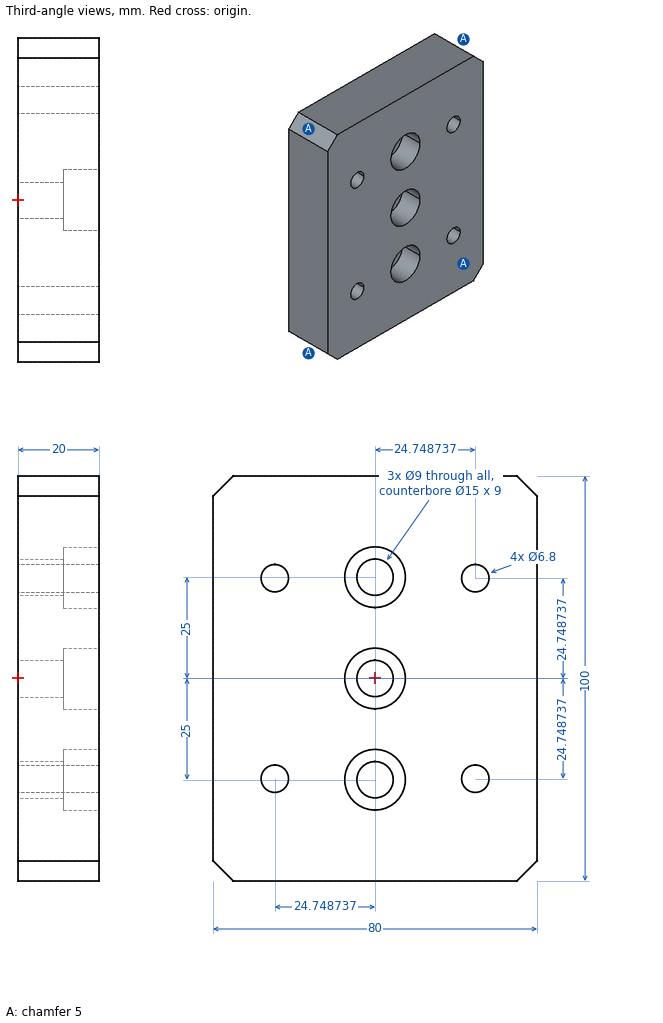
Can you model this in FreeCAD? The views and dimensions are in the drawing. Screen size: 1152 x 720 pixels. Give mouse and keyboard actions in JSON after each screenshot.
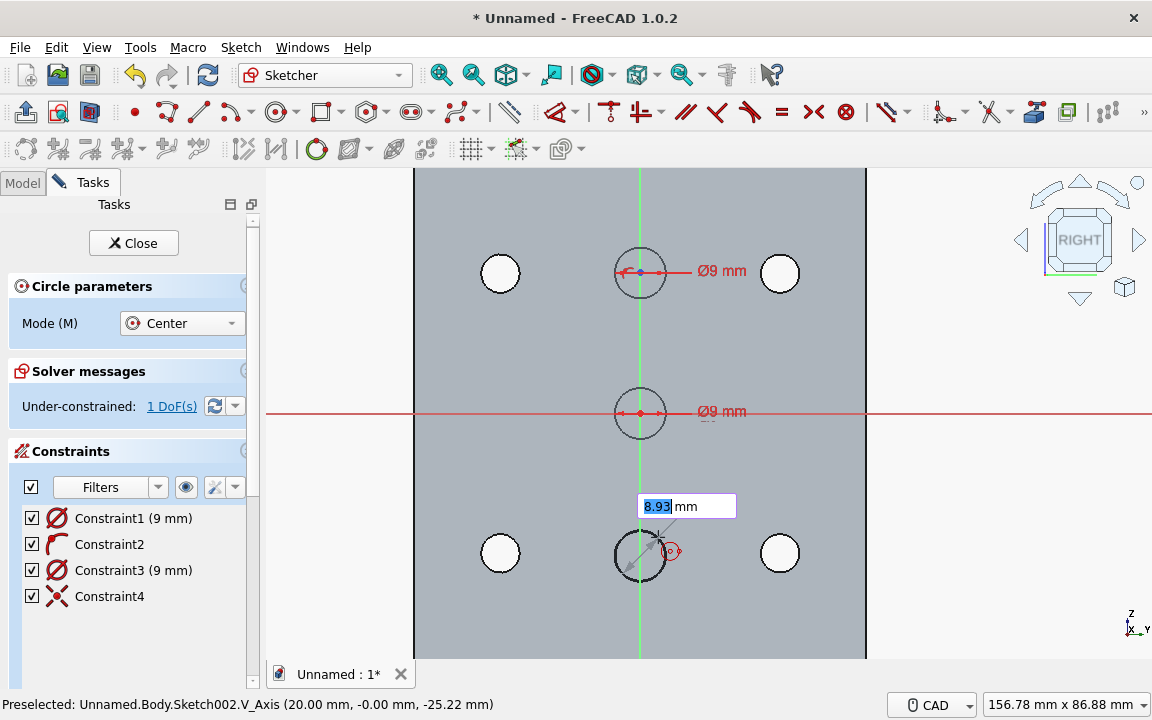
{"action": "type", "text": "9"}
{"action": "key", "text": "Return"}
{"action": "key", "text": "Escape"}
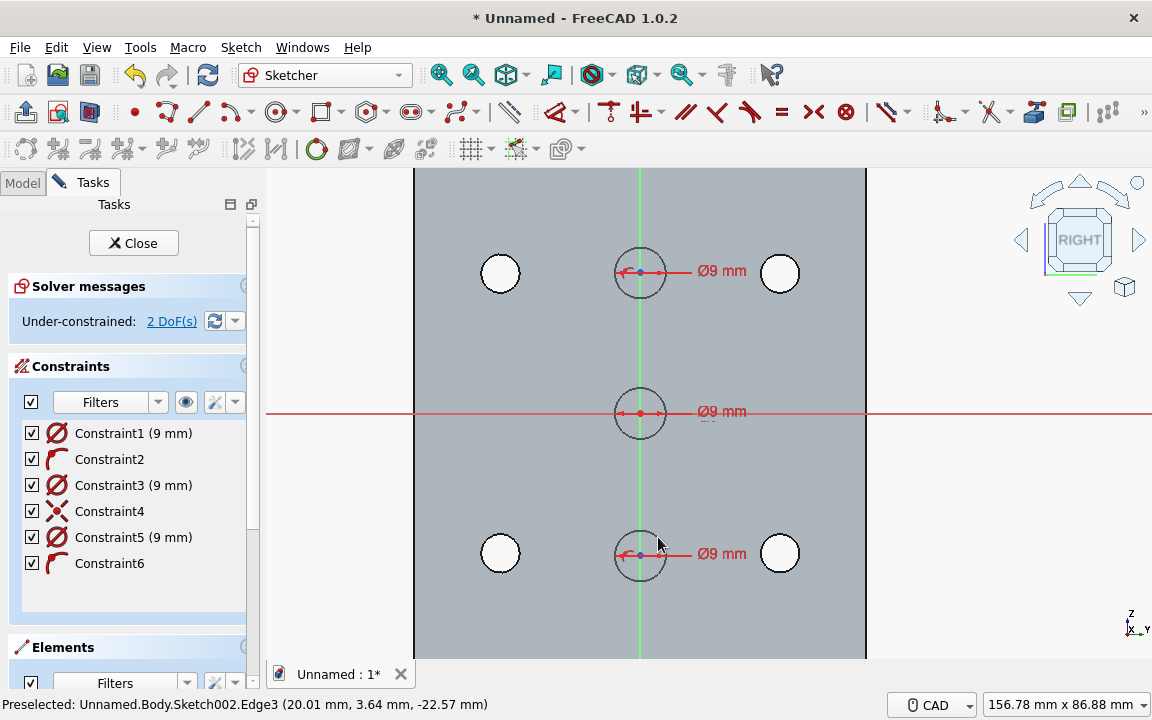
{"action": "key", "text": "d"}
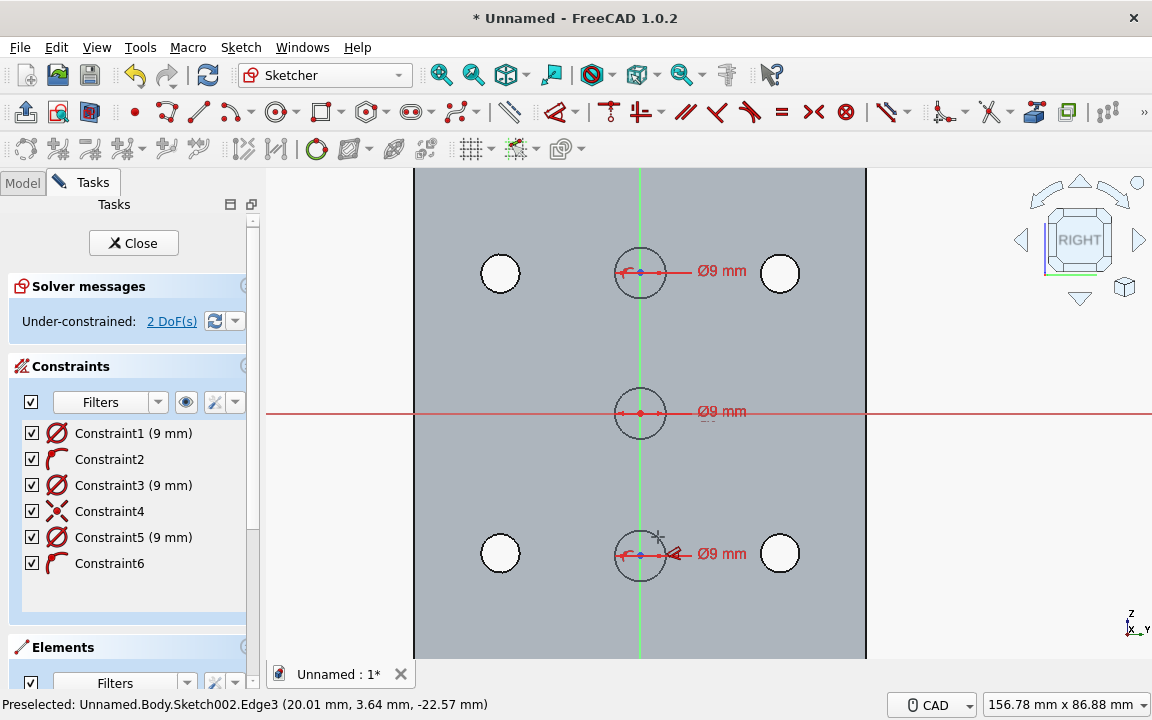
{"action": "left_click", "coordinate": [640, 273]}
{"action": "left_click", "coordinate": [674, 343]}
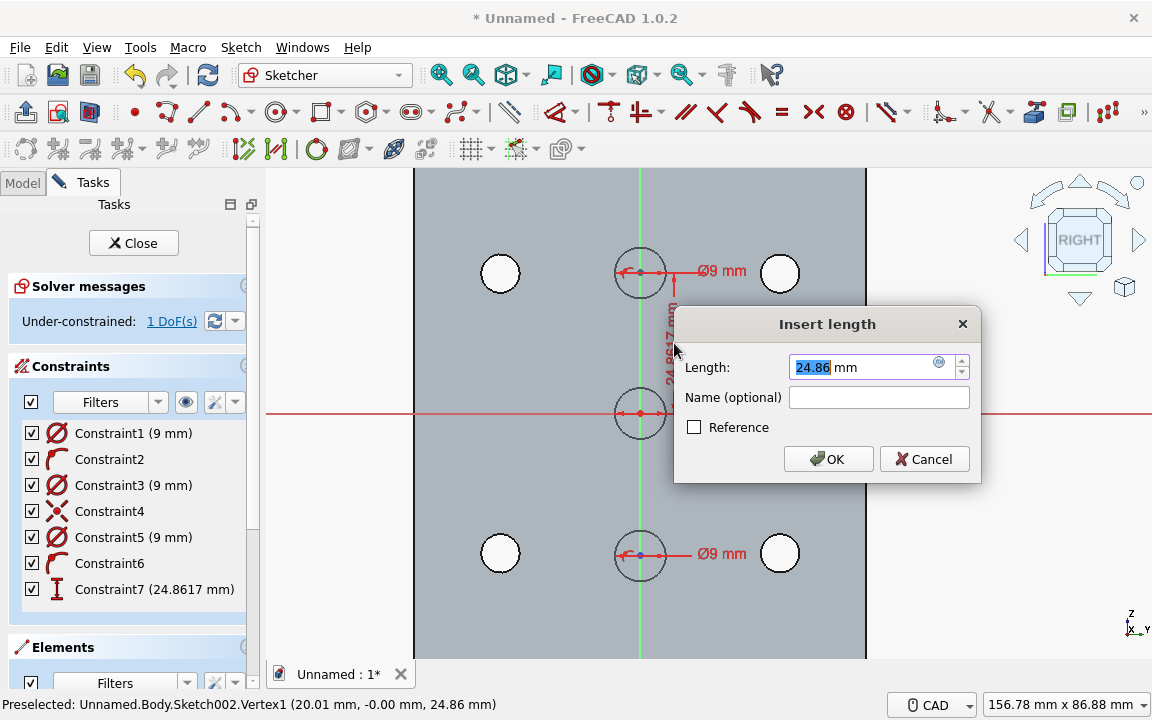
{"action": "type", "text": "25"}
{"action": "key", "text": "Return"}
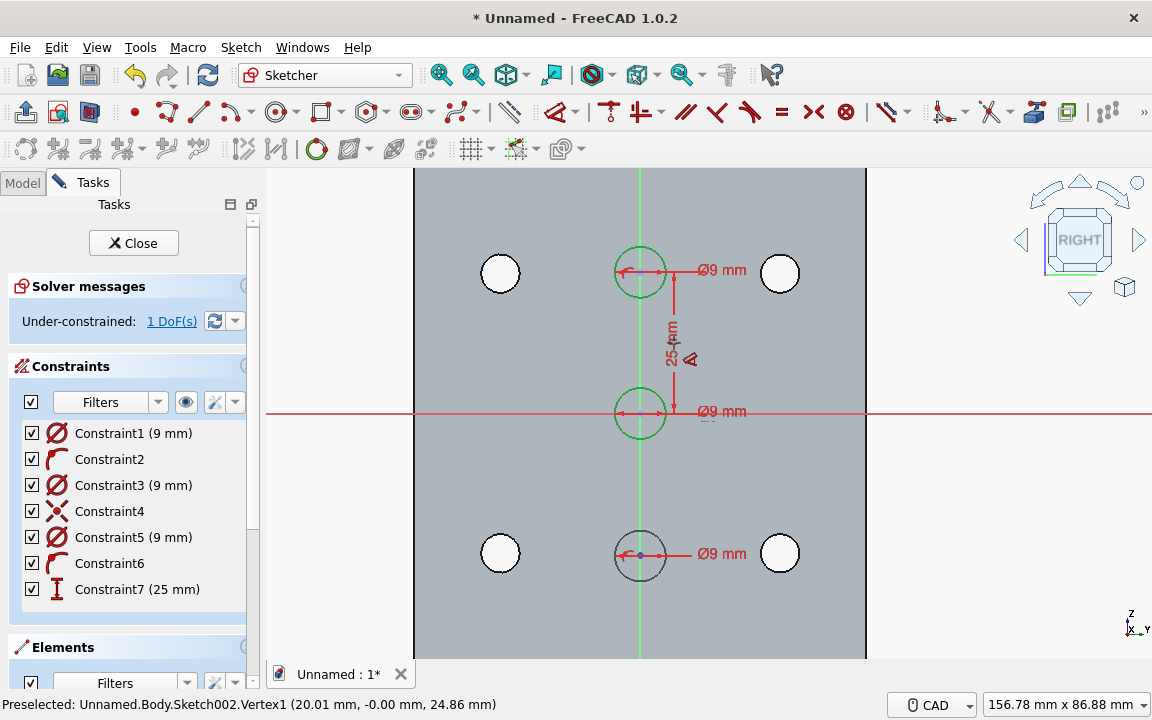
{"action": "left_click", "coordinate": [640, 556]}
{"action": "left_click", "coordinate": [674, 485]}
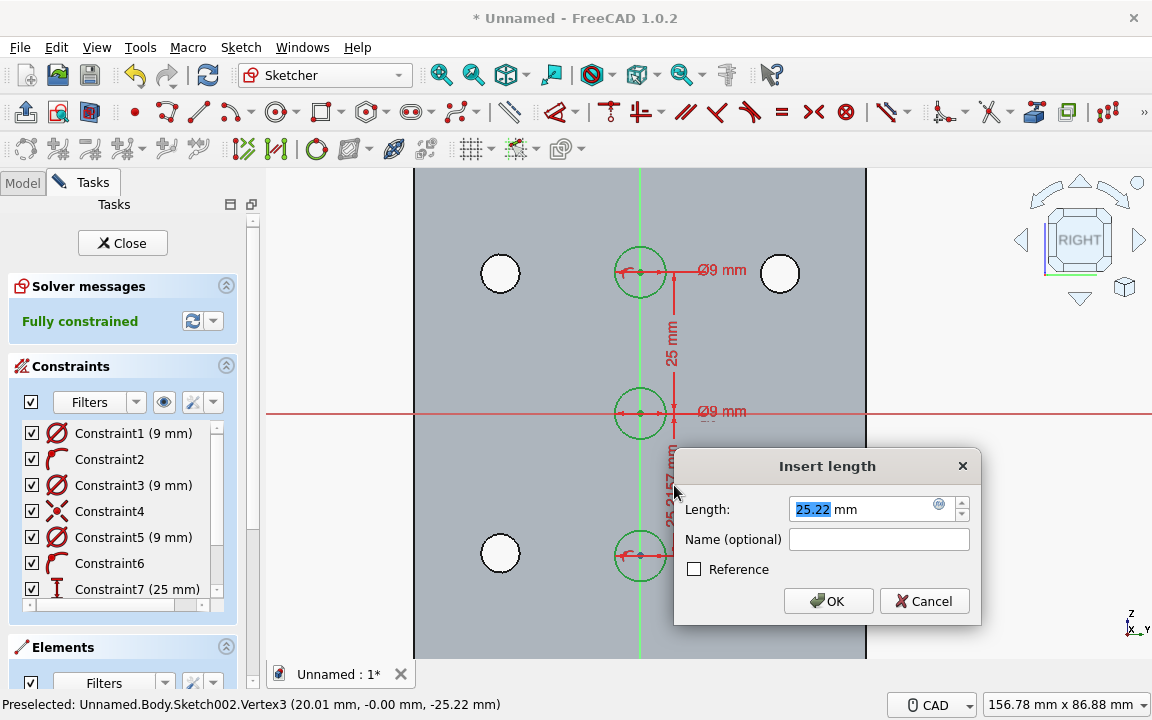
{"action": "type", "text": "25"}
{"action": "key", "text": "Return"}
{"action": "key", "text": "Escape"}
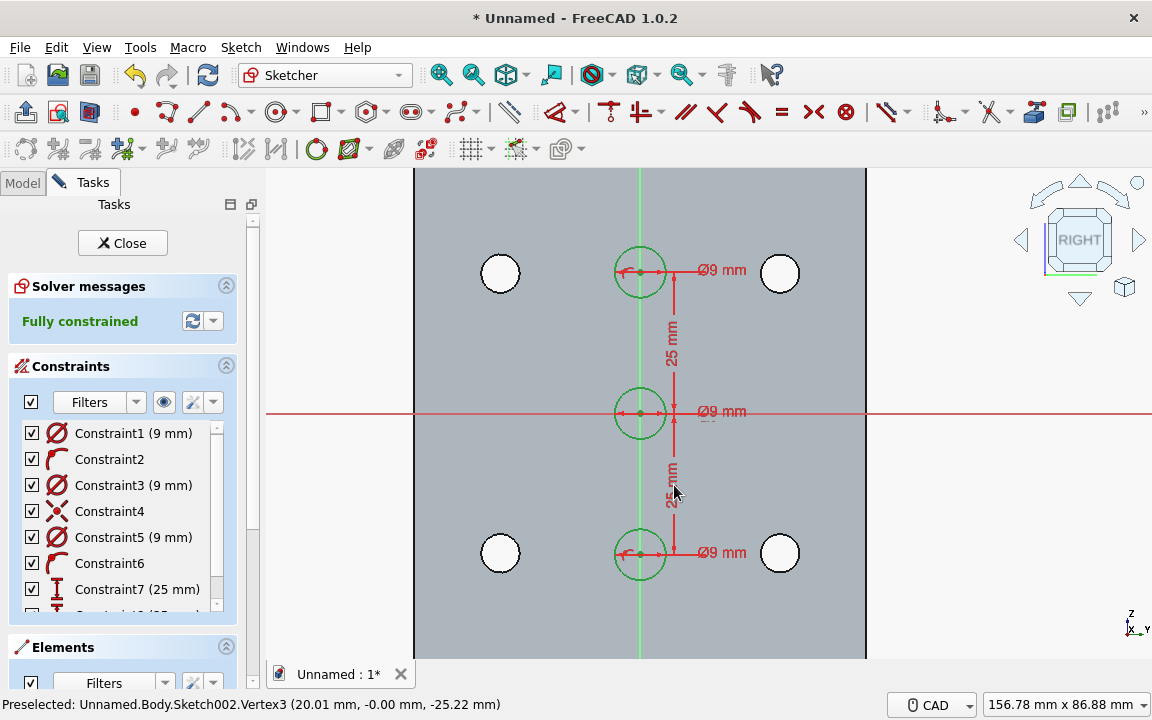
{"action": "left_click", "coordinate": [123, 243]}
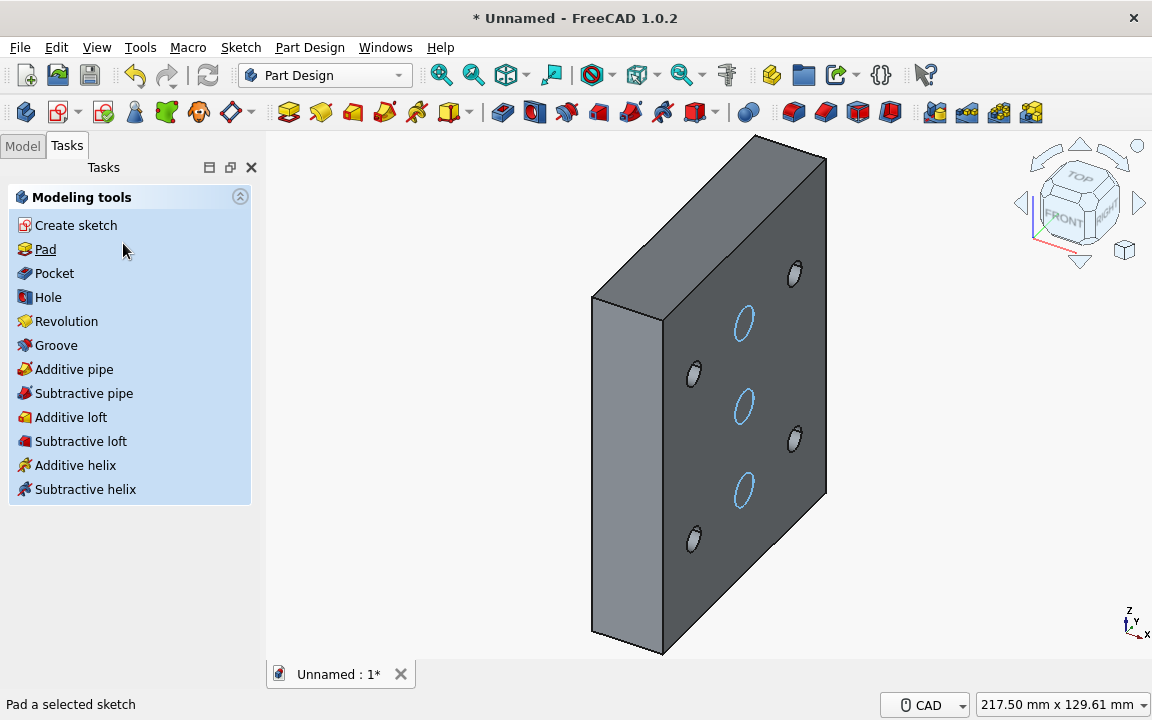
{"action": "left_click", "coordinate": [536, 112]}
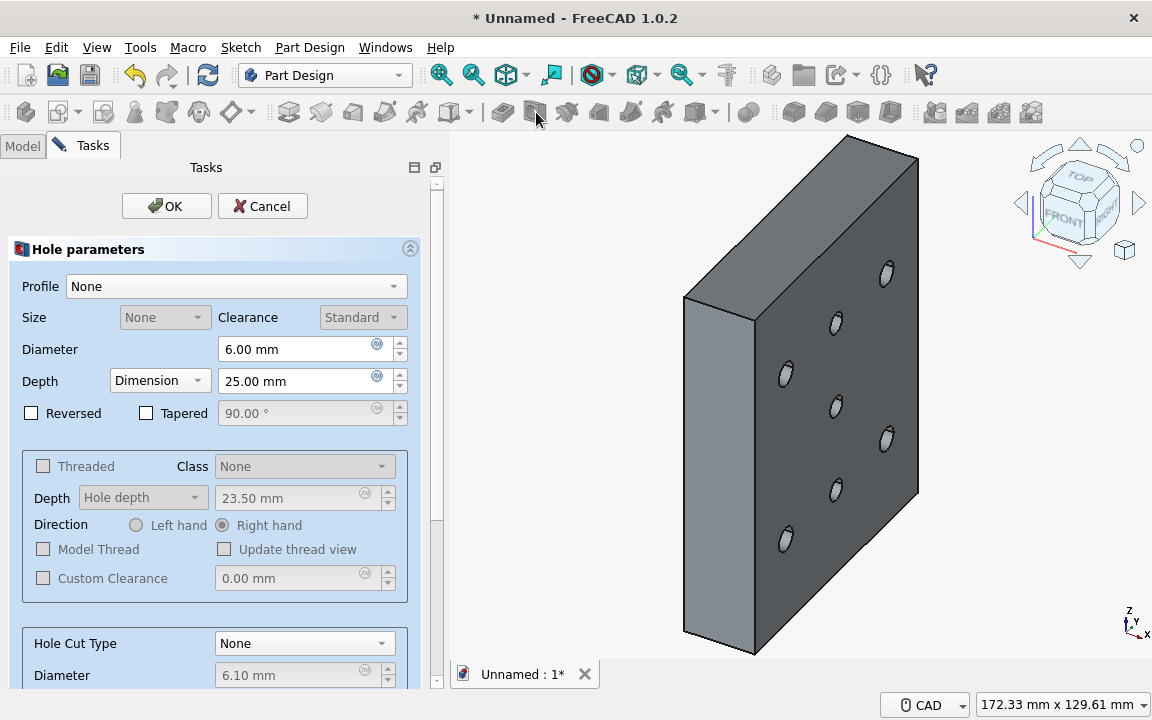
{"action": "triple_click", "coordinate": [305, 349]}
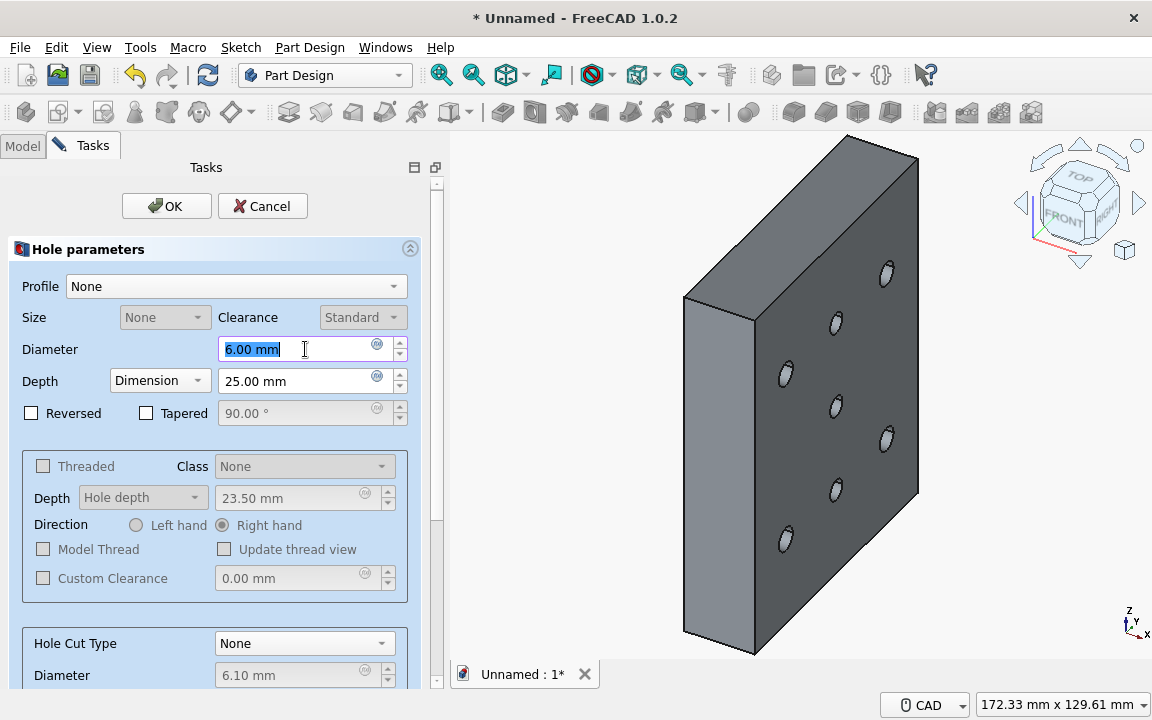
{"action": "type", "text": "9"}
{"action": "key", "text": "Tab"}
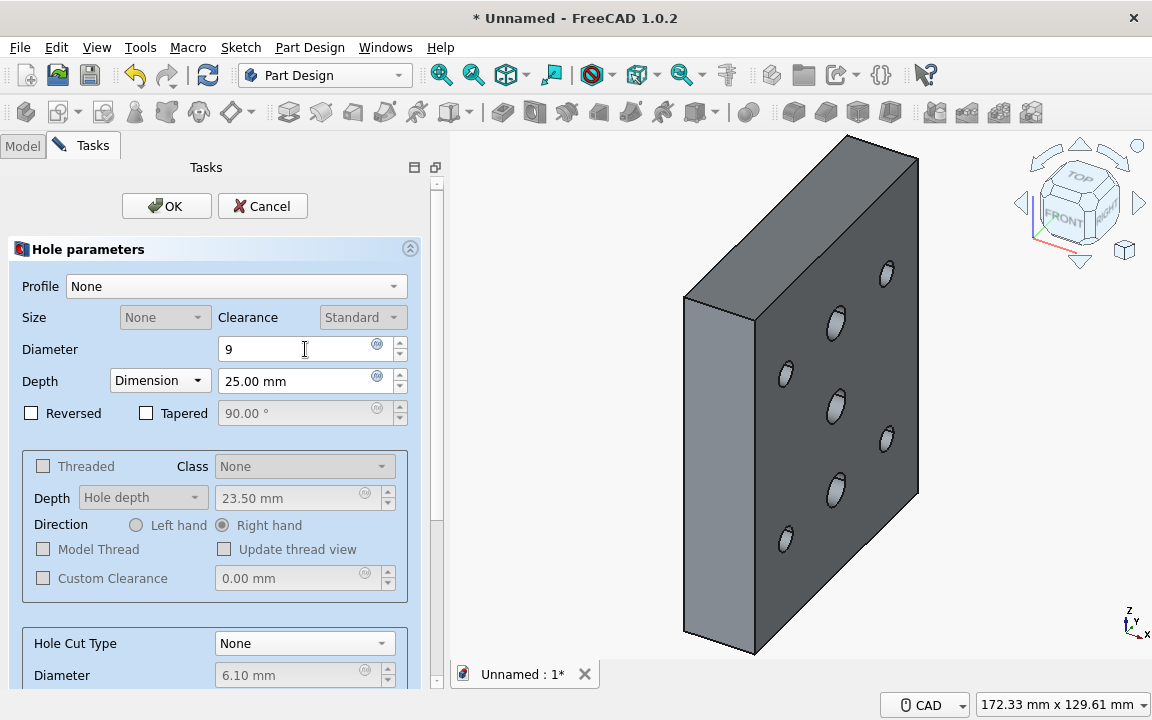
{"action": "left_click", "coordinate": [161, 380]}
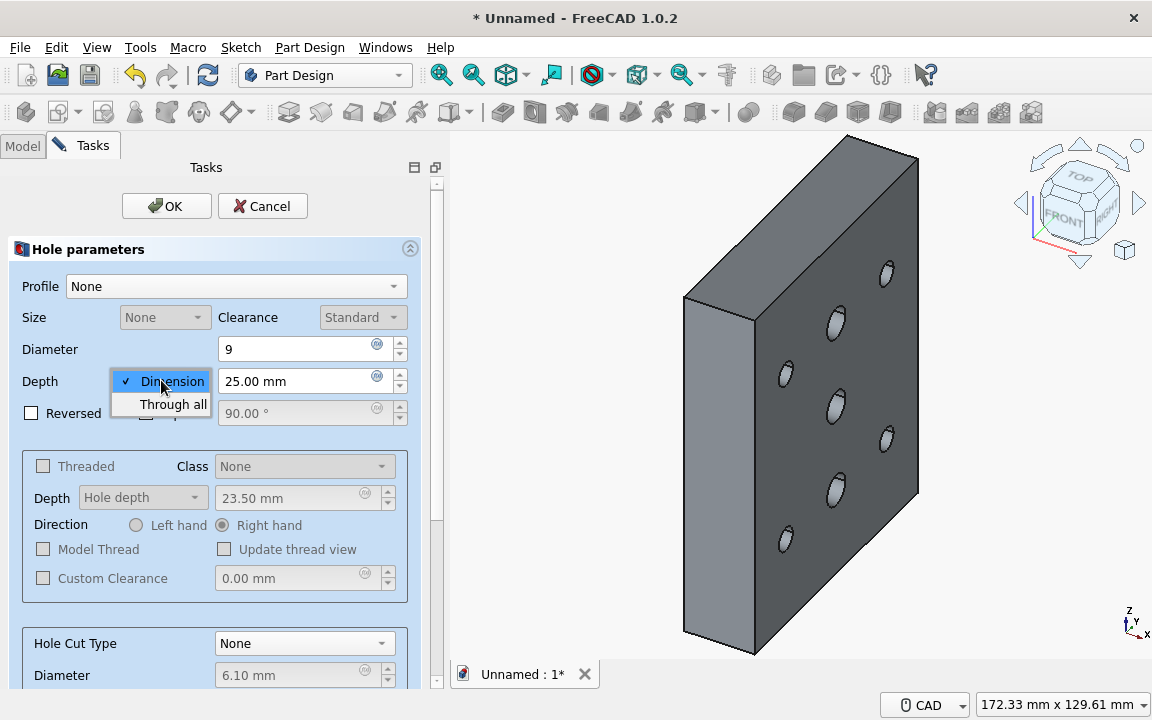
{"action": "left_click", "coordinate": [160, 404]}